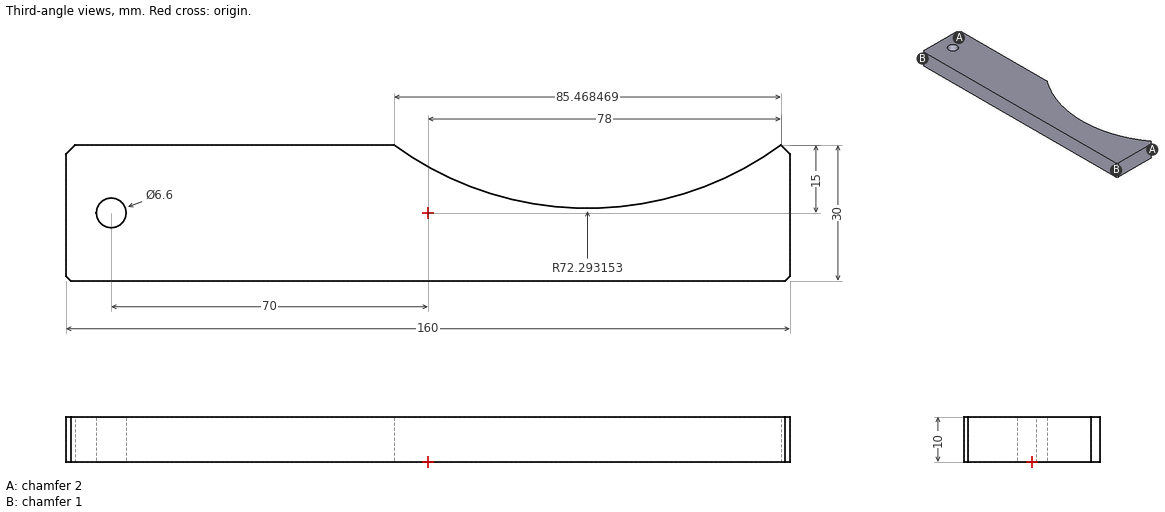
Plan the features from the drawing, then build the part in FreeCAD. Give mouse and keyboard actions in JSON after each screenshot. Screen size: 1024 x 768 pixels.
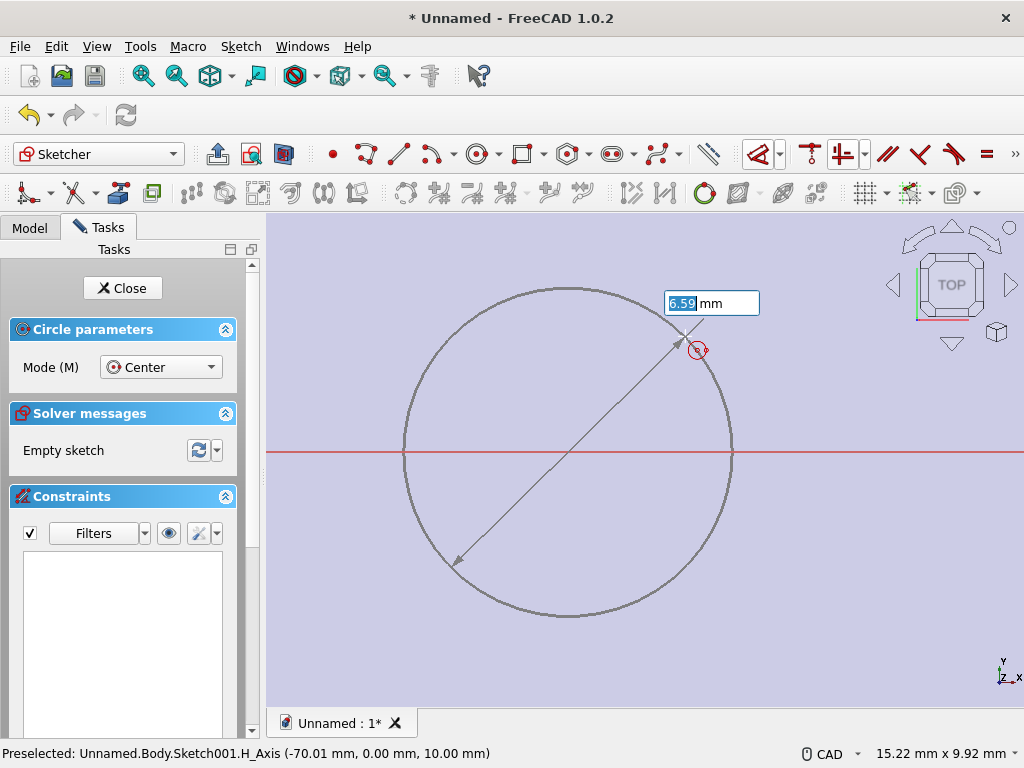
{"action": "type", "text": "6.6"}
{"action": "key", "text": "Return"}
{"action": "key", "text": "Escape"}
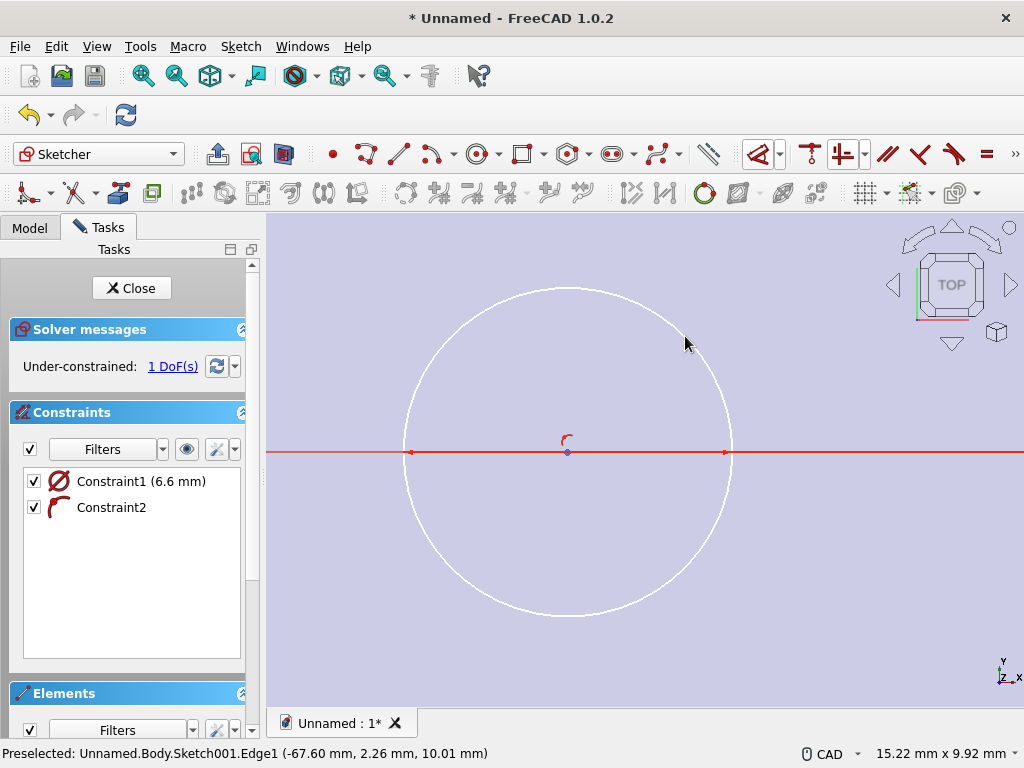
{"action": "key", "text": "d"}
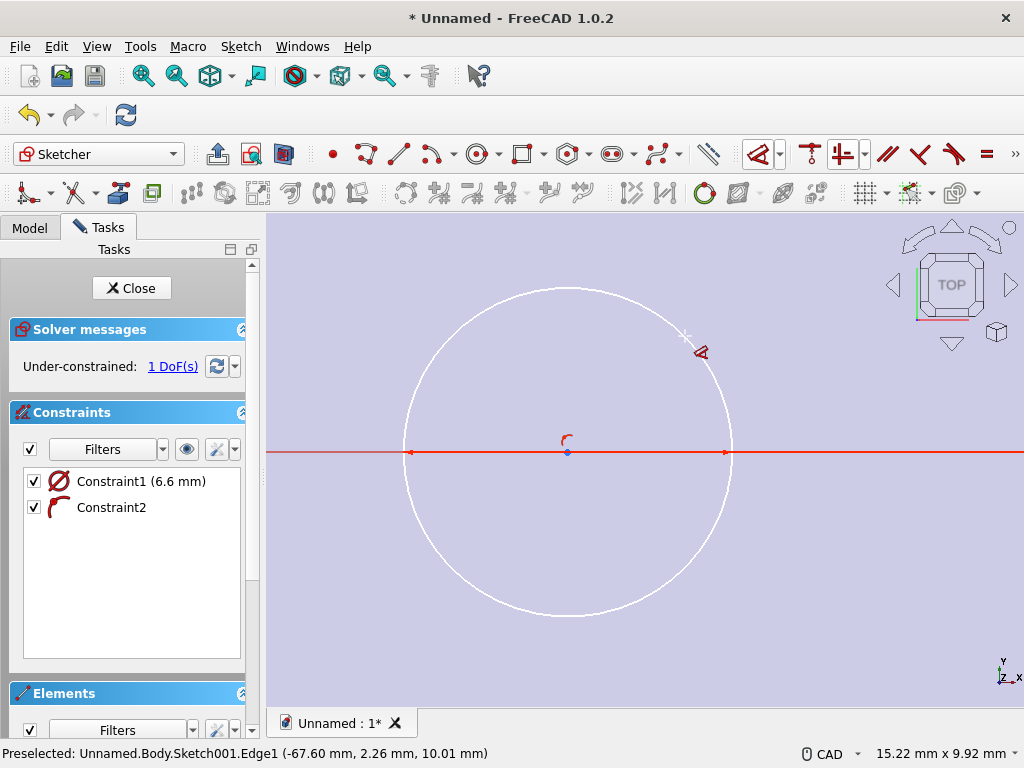
{"action": "left_click", "coordinate": [568, 452]}
{"action": "left_click", "coordinate": [713, 486]}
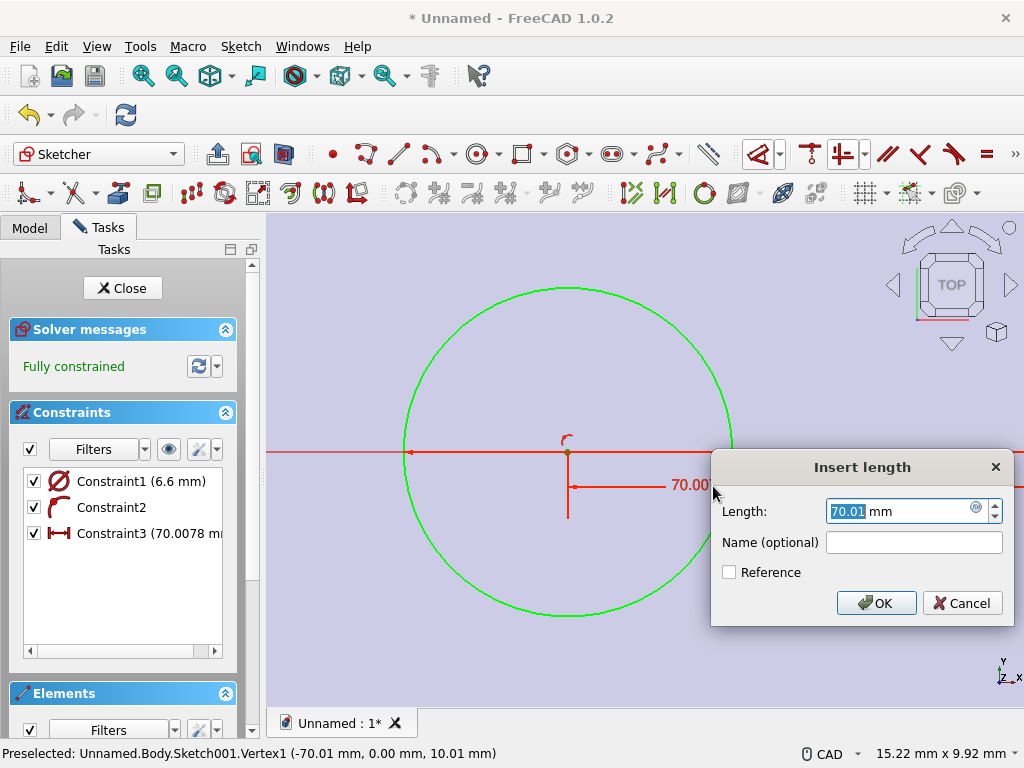
{"action": "type", "text": "70"}
{"action": "key", "text": "Return"}
{"action": "key", "text": "Escape"}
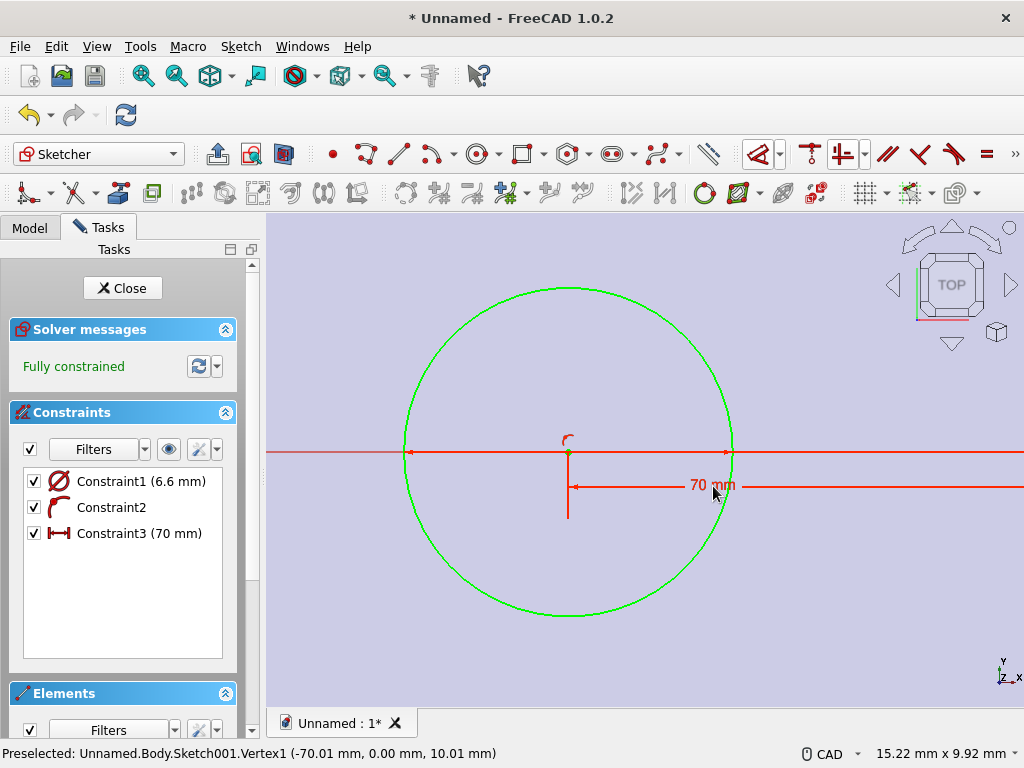
{"action": "left_click", "coordinate": [123, 288]}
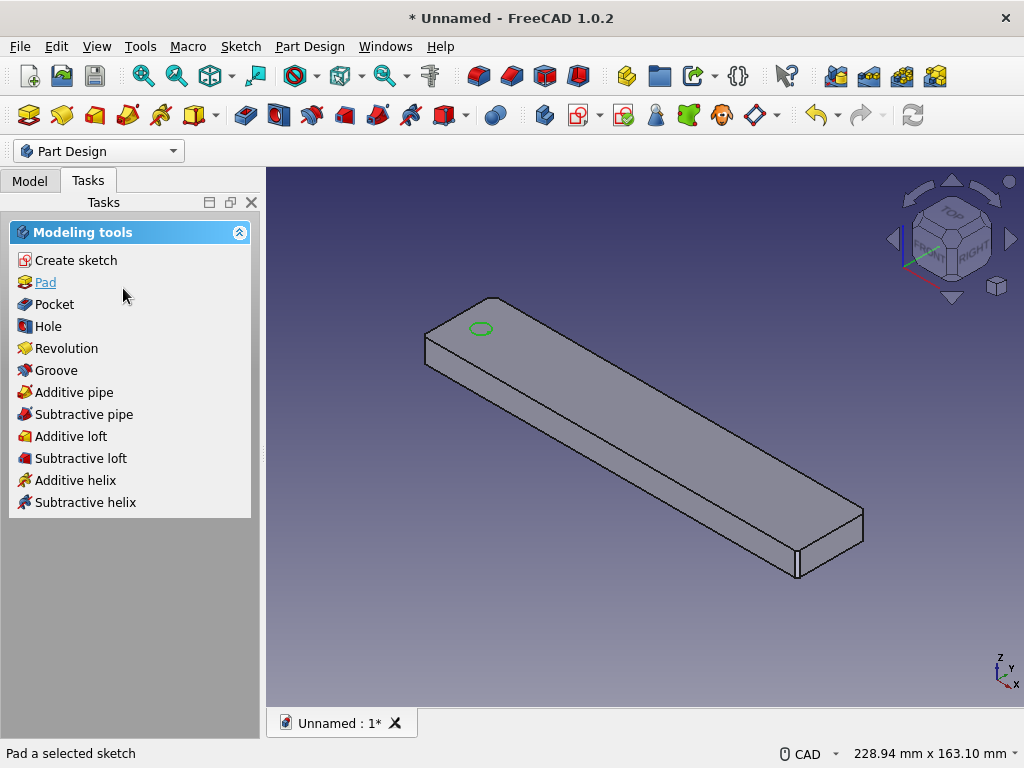
{"action": "left_click", "coordinate": [246, 116]}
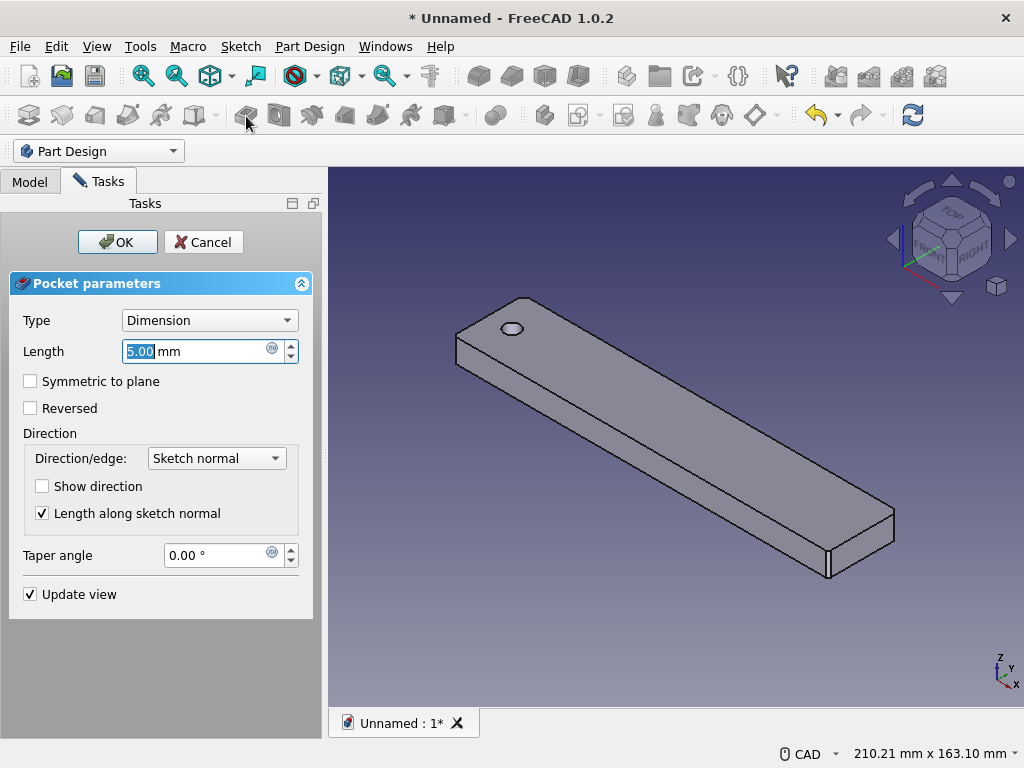
{"action": "left_click", "coordinate": [210, 320]}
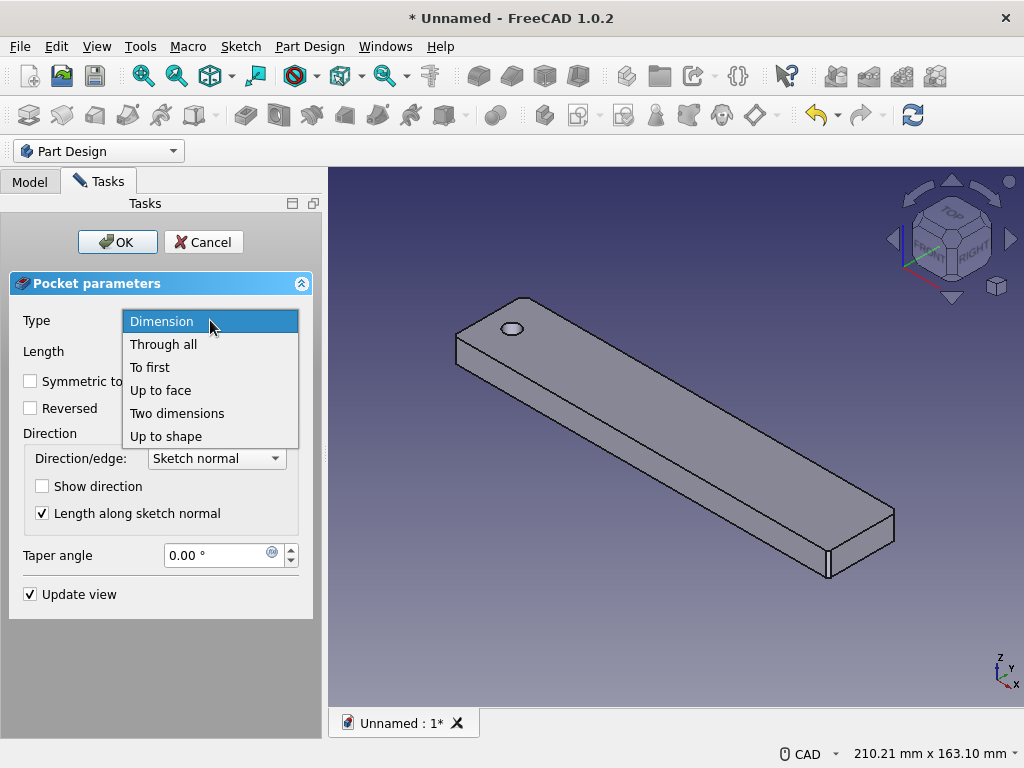
{"action": "left_click", "coordinate": [208, 344]}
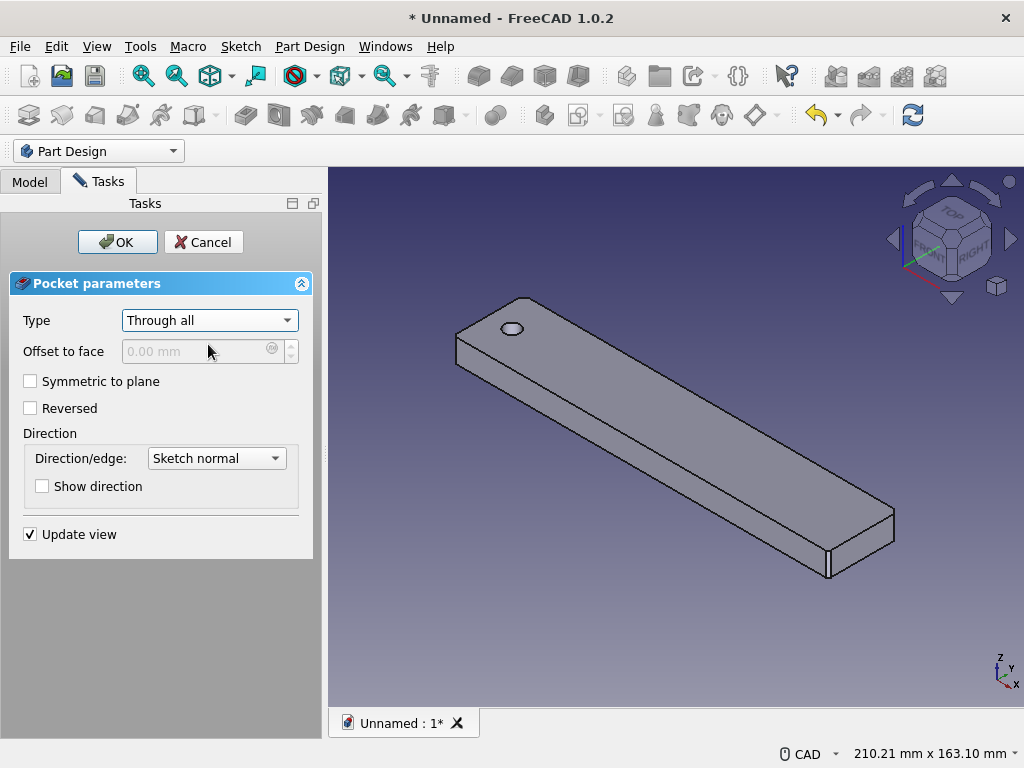
{"action": "left_click", "coordinate": [118, 242]}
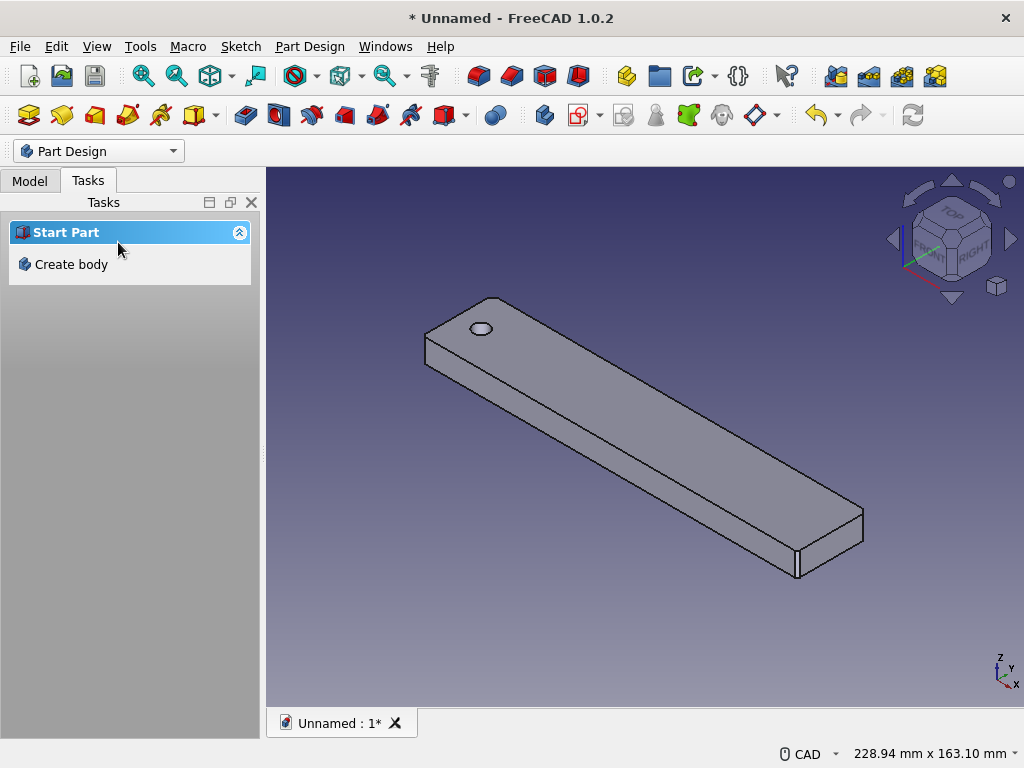
{"action": "left_click", "coordinate": [752, 484]}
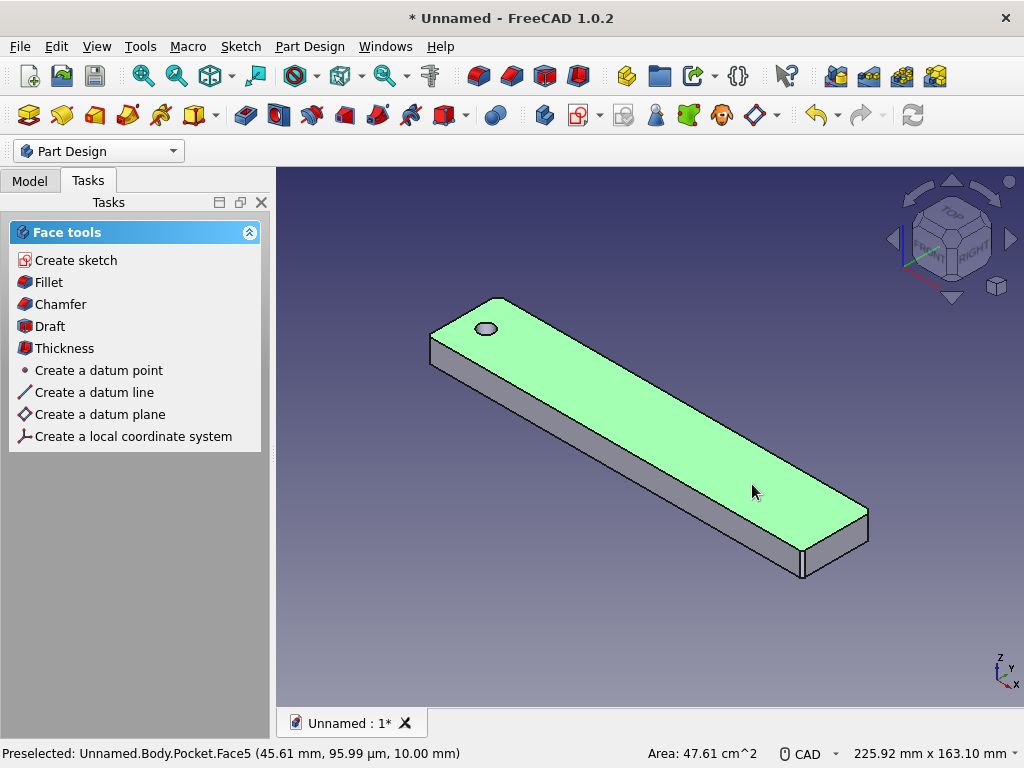
{"action": "left_click", "coordinate": [578, 116]}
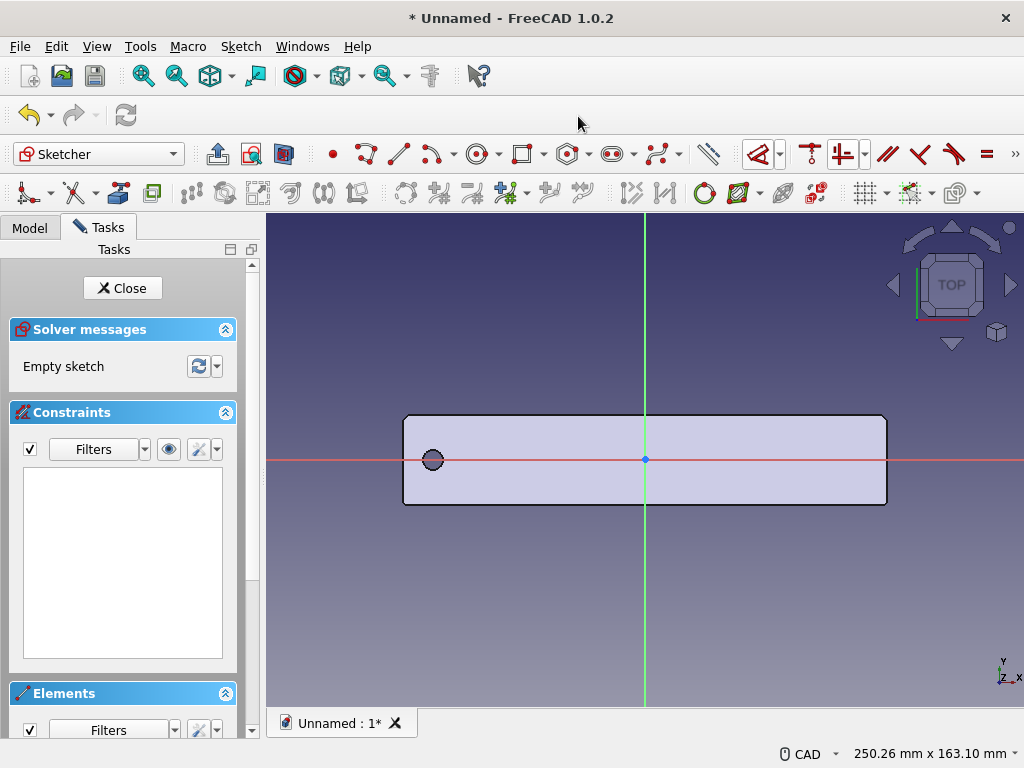
{"action": "scroll", "coordinate": [294, 563], "scroll_direction": "down", "scroll_amount": 1}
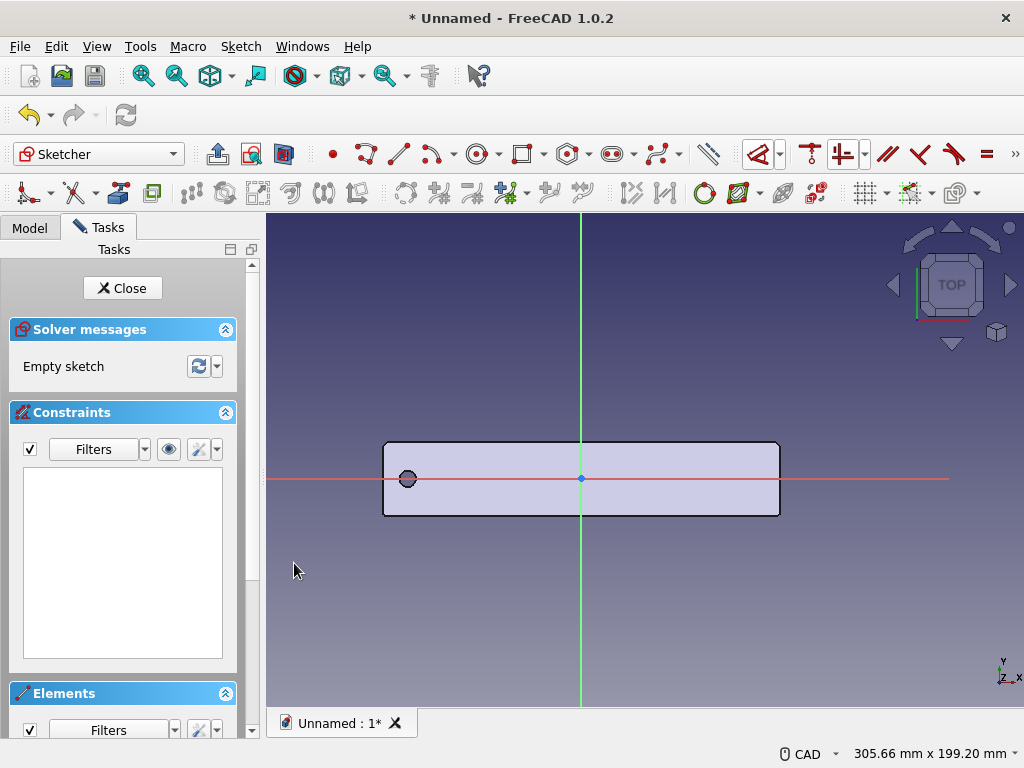
{"action": "scroll", "coordinate": [781, 460], "scroll_direction": "up", "scroll_amount": 3}